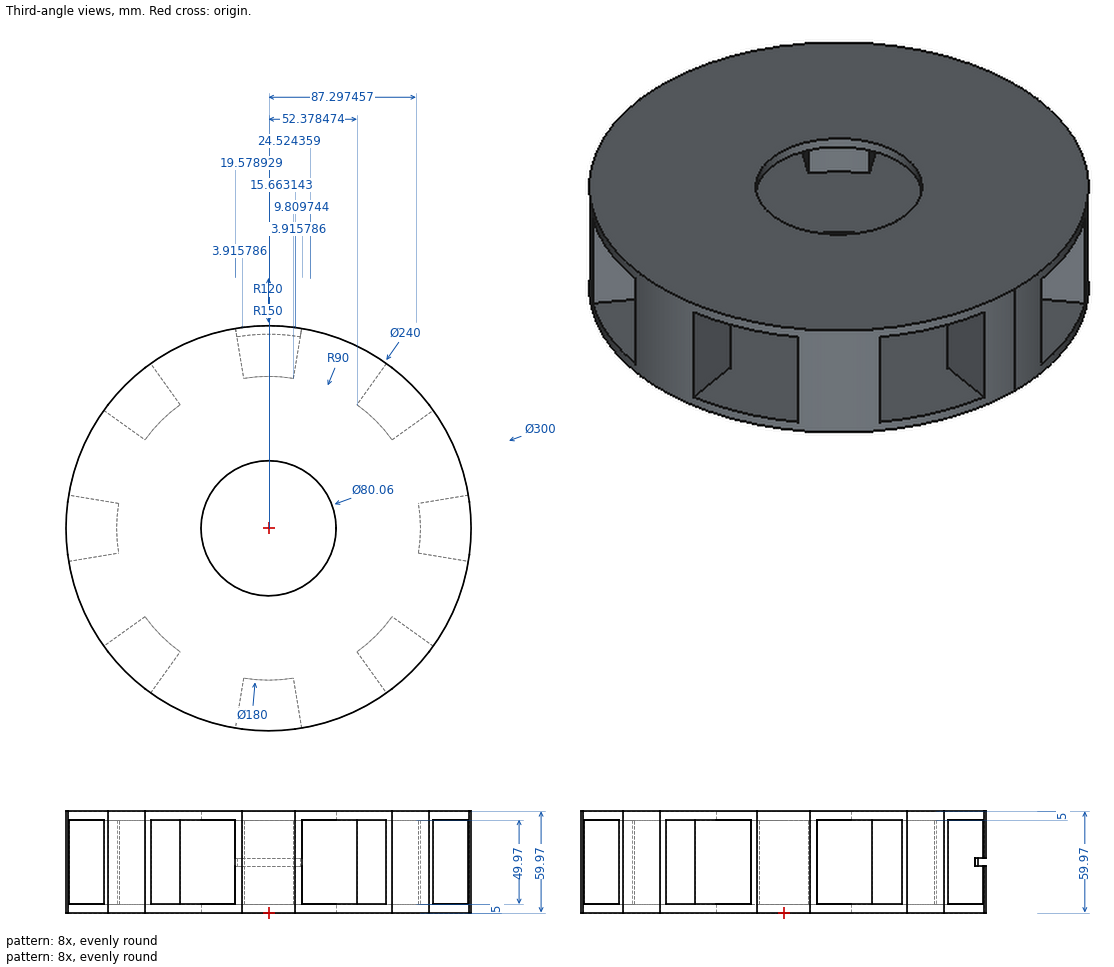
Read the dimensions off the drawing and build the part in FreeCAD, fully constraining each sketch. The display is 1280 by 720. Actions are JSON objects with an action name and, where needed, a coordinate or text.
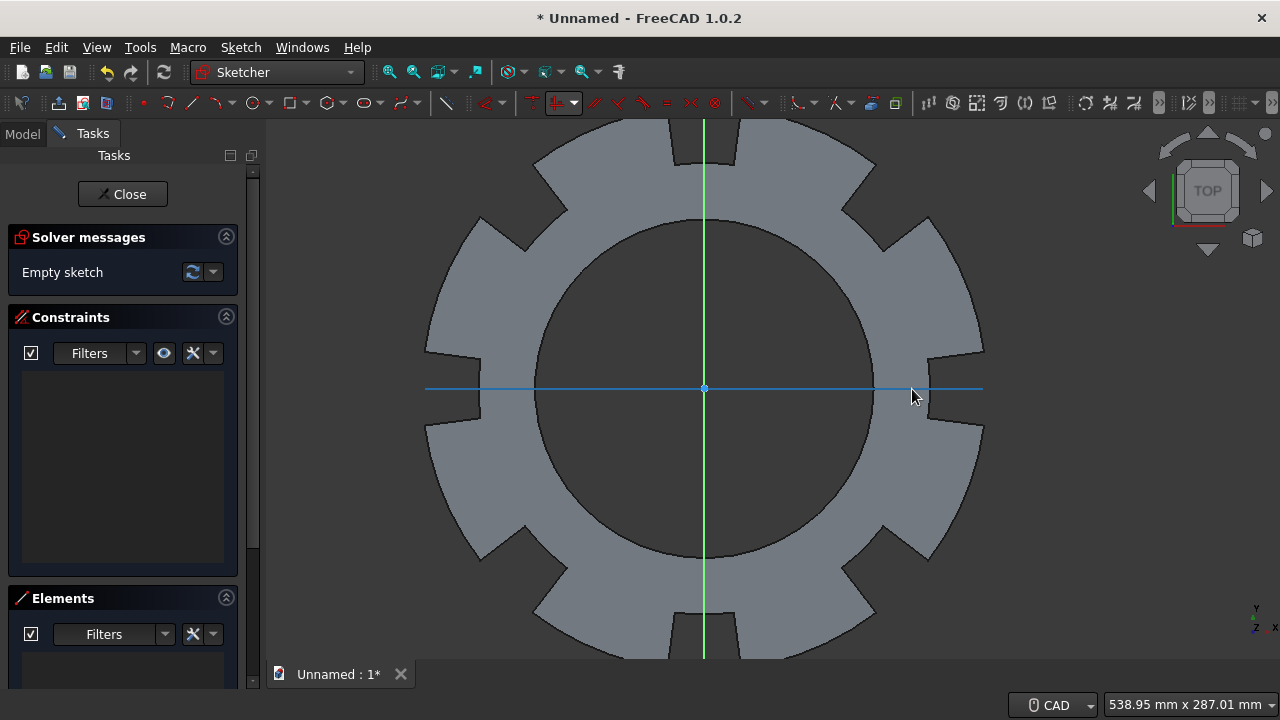
{"action": "key", "text": "g c"}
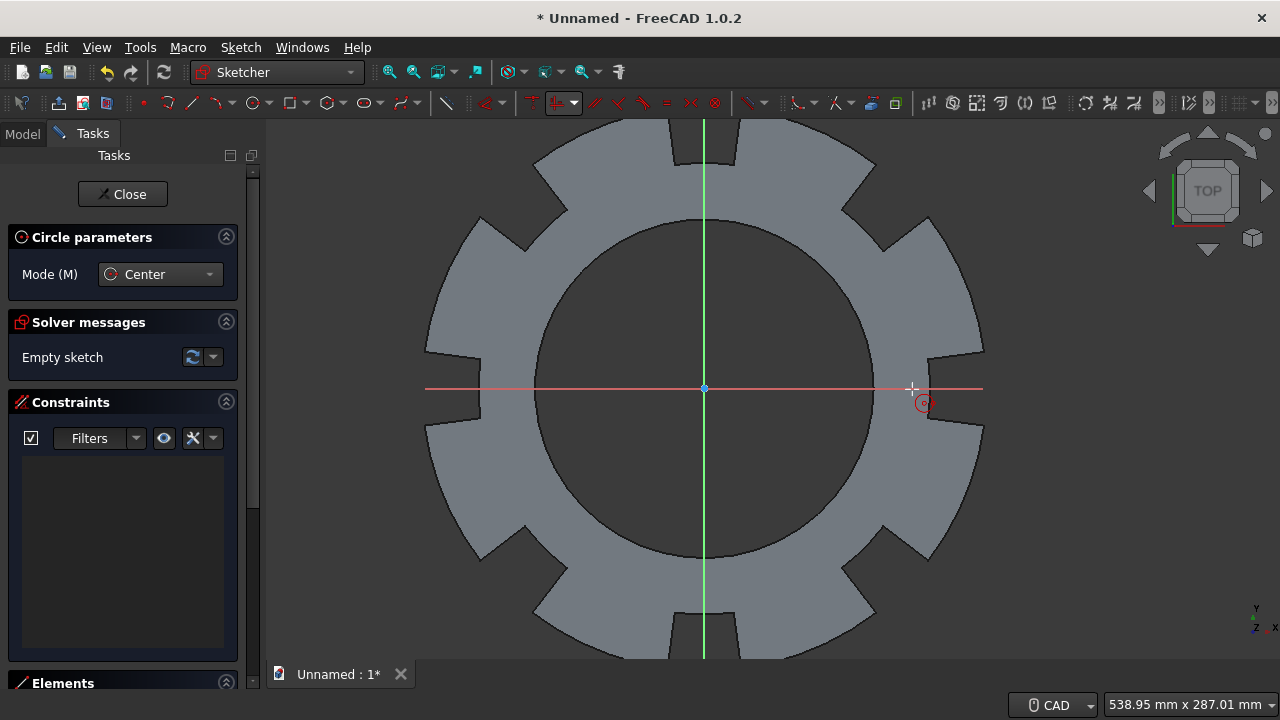
{"action": "left_click", "coordinate": [704, 389]}
{"action": "left_click", "coordinate": [824, 269]}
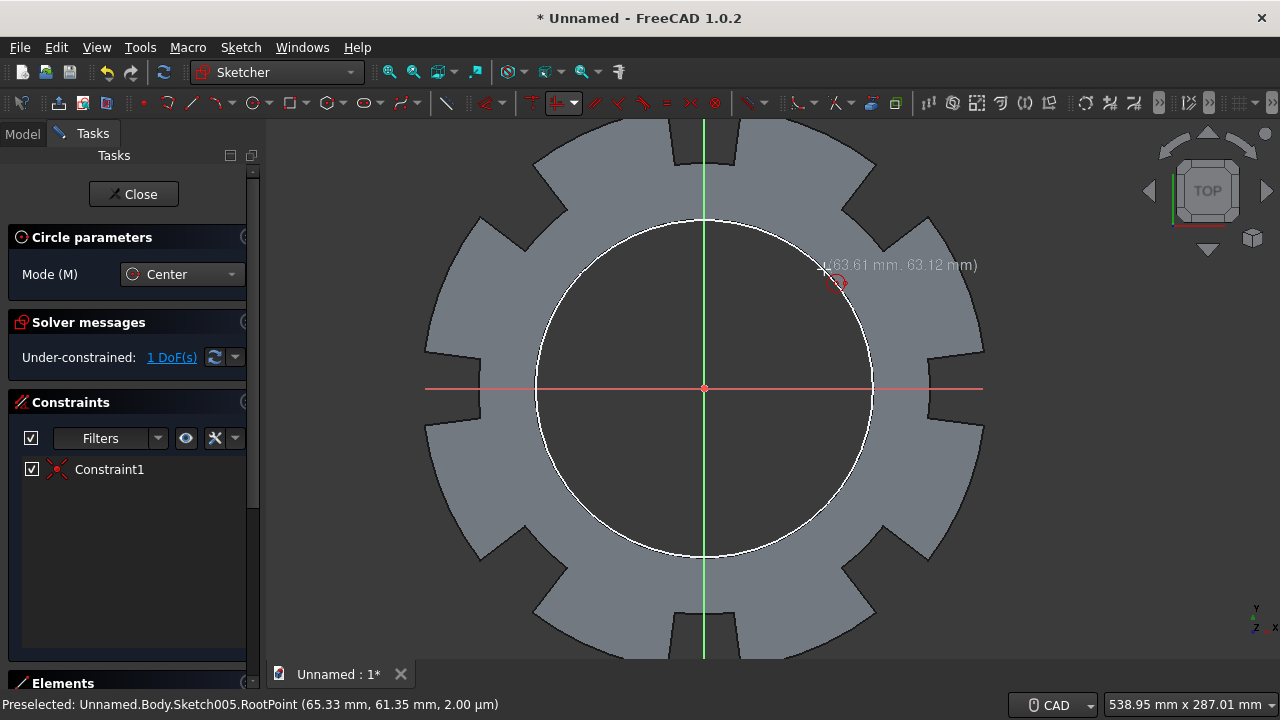
{"action": "left_click", "coordinate": [704, 389]}
{"action": "left_click", "coordinate": [758, 335]}
{"action": "key", "text": "Escape"}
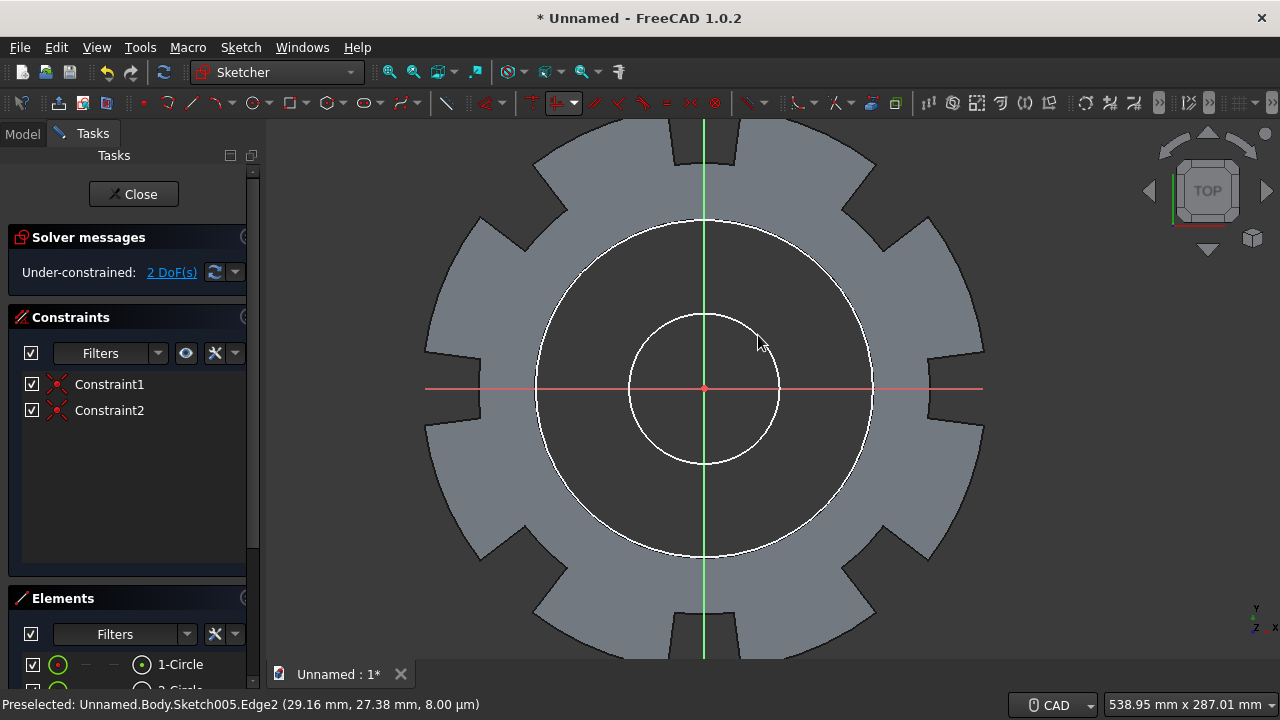
{"action": "left_click", "coordinate": [486, 104]}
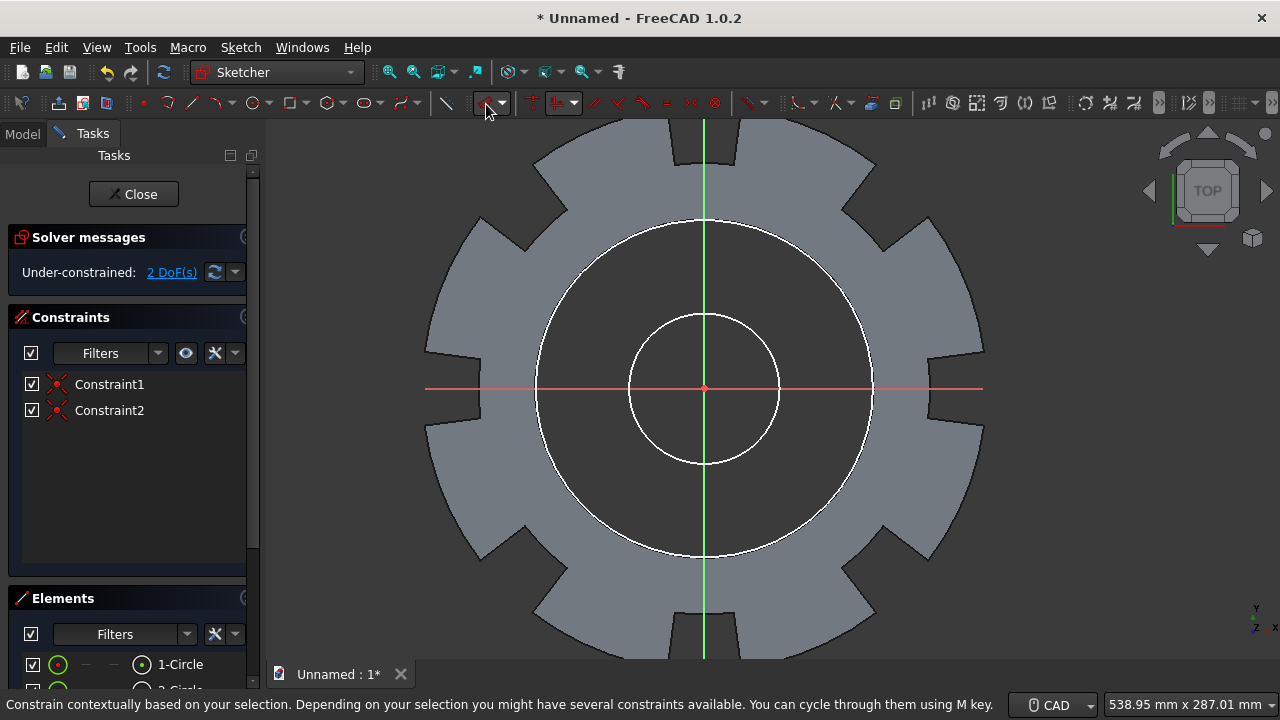
{"action": "left_click", "coordinate": [823, 269]}
{"action": "left_click", "coordinate": [846, 246]}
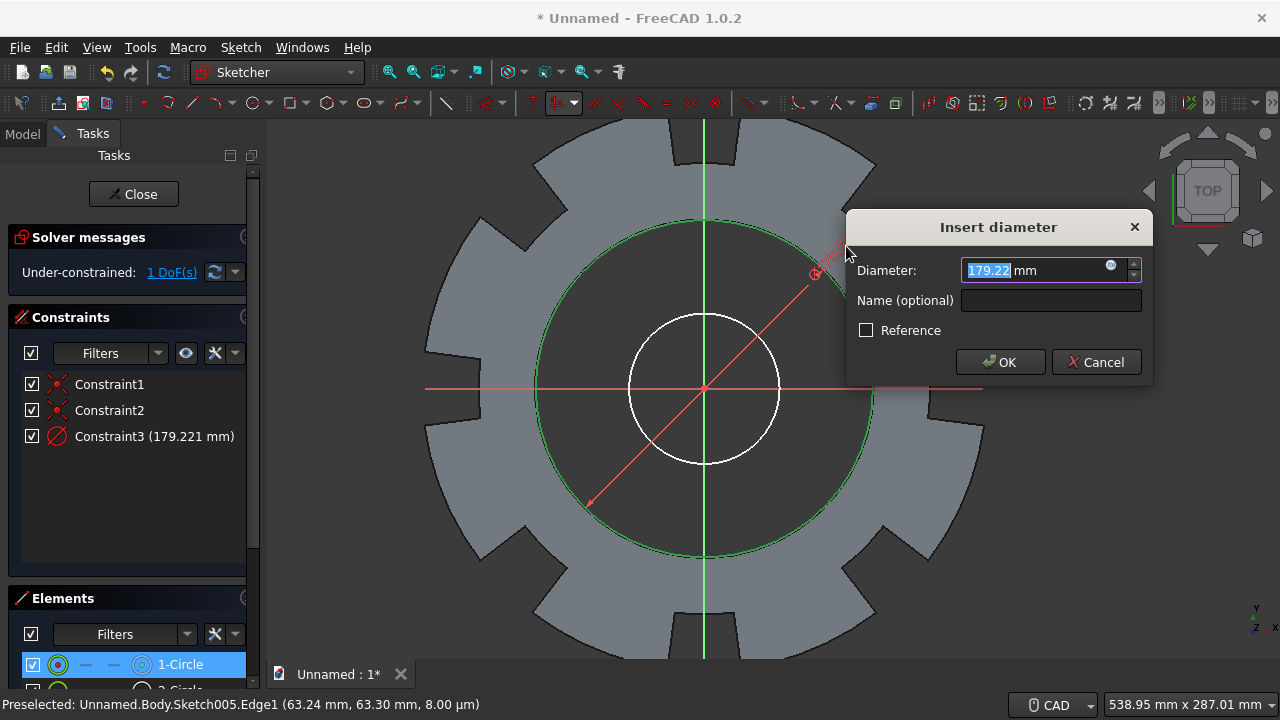
{"action": "type", "text": "180"}
{"action": "key", "text": "Return"}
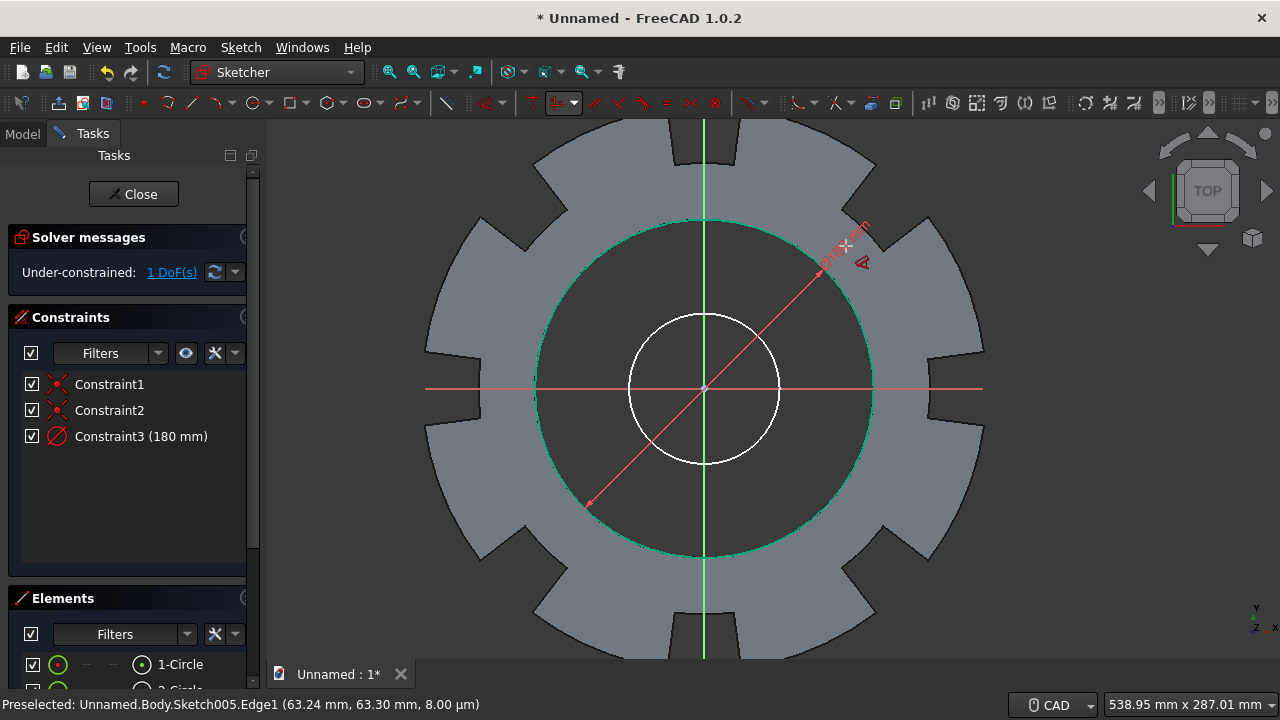
{"action": "left_click", "coordinate": [757, 335]}
{"action": "left_click", "coordinate": [779, 312]}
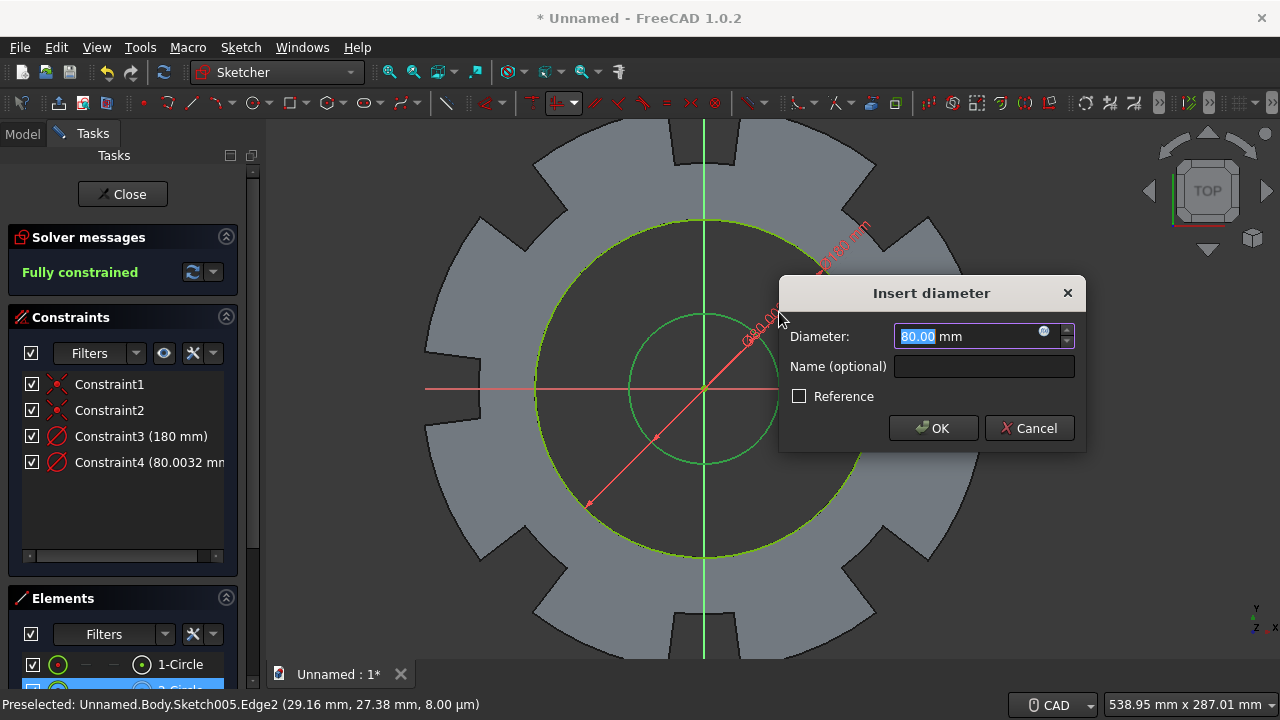
{"action": "type", "text": "80.06"}
{"action": "key", "text": "Return"}
{"action": "key", "text": "Escape"}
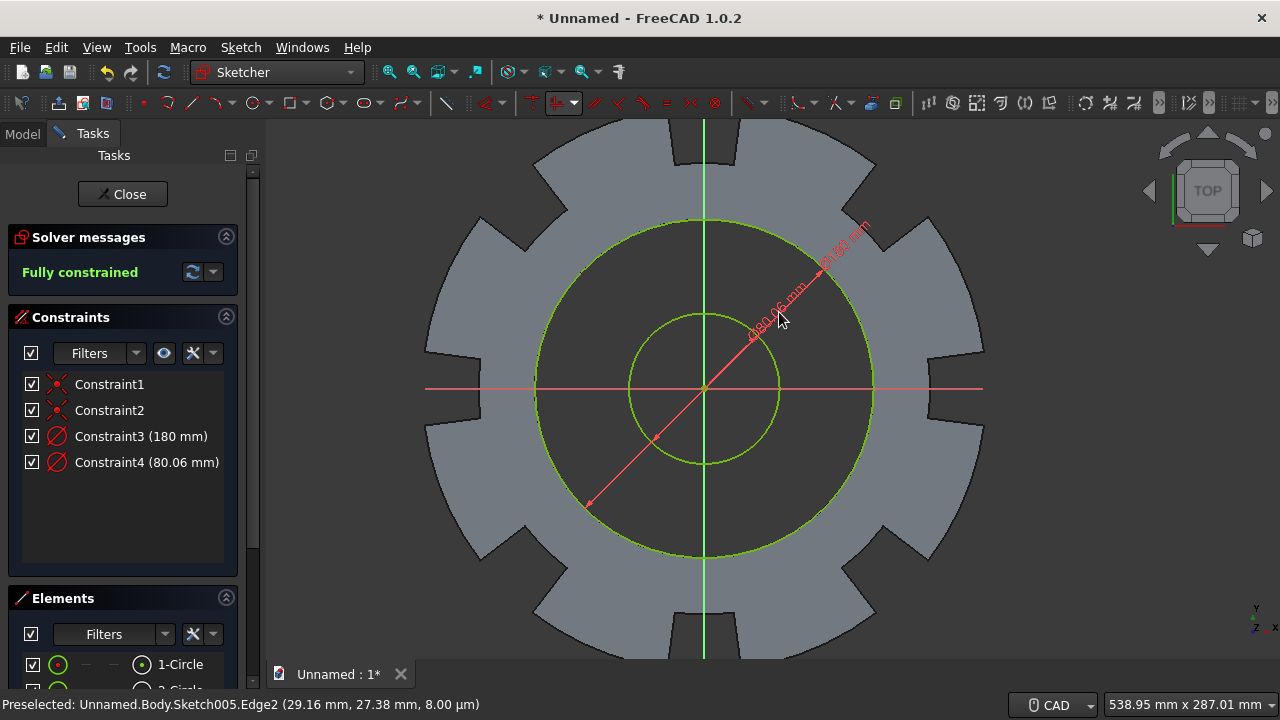
{"action": "left_click", "coordinate": [123, 194]}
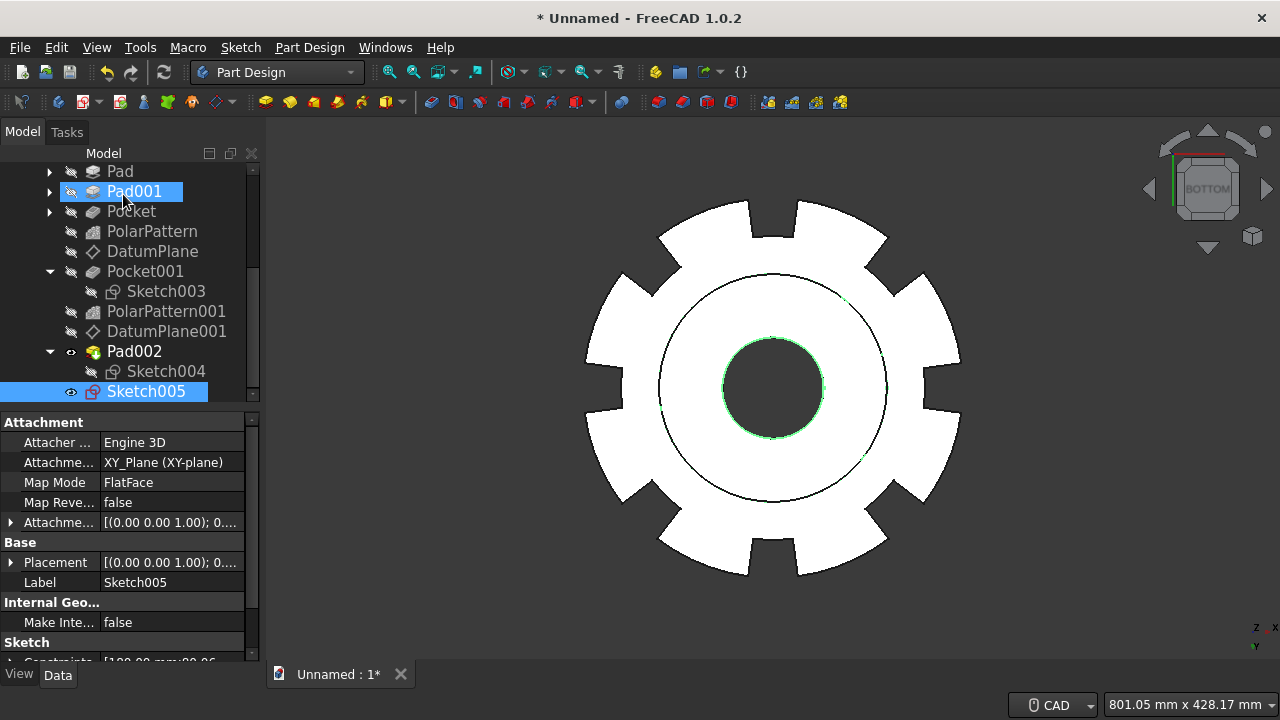
{"action": "left_click", "coordinate": [266, 102]}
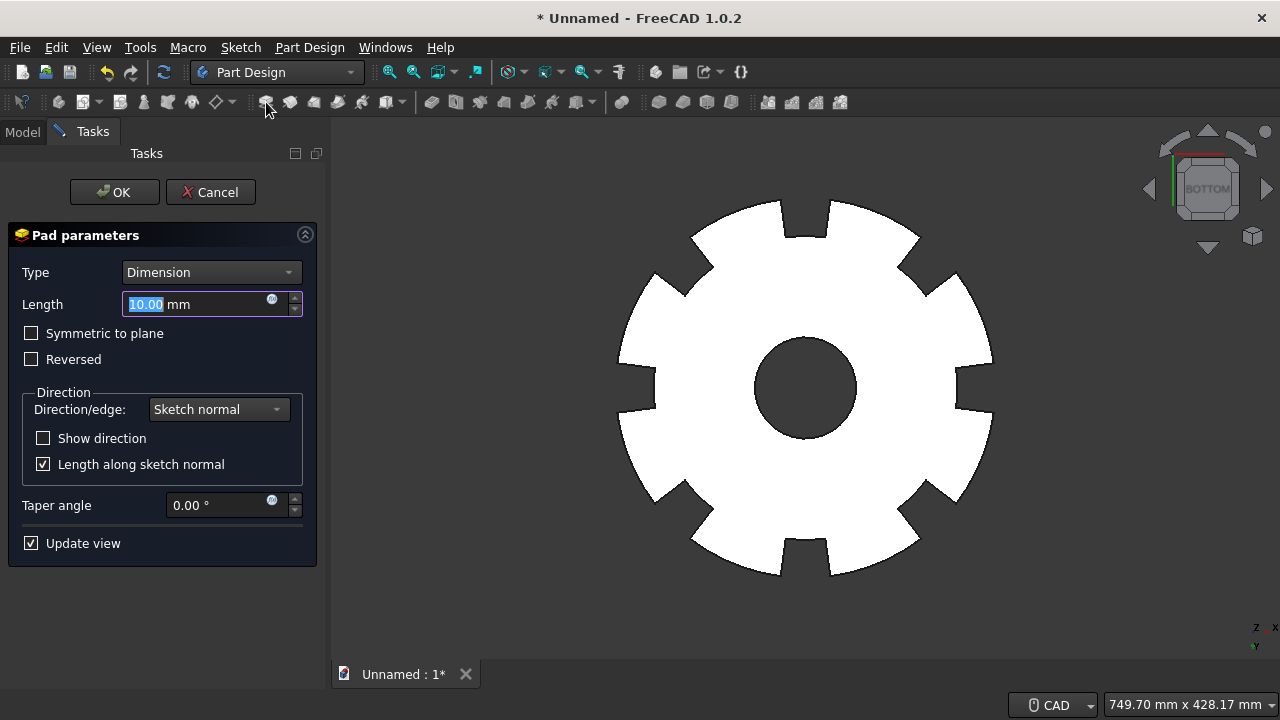
{"action": "type", "text": "5"}
{"action": "key", "text": "Tab"}